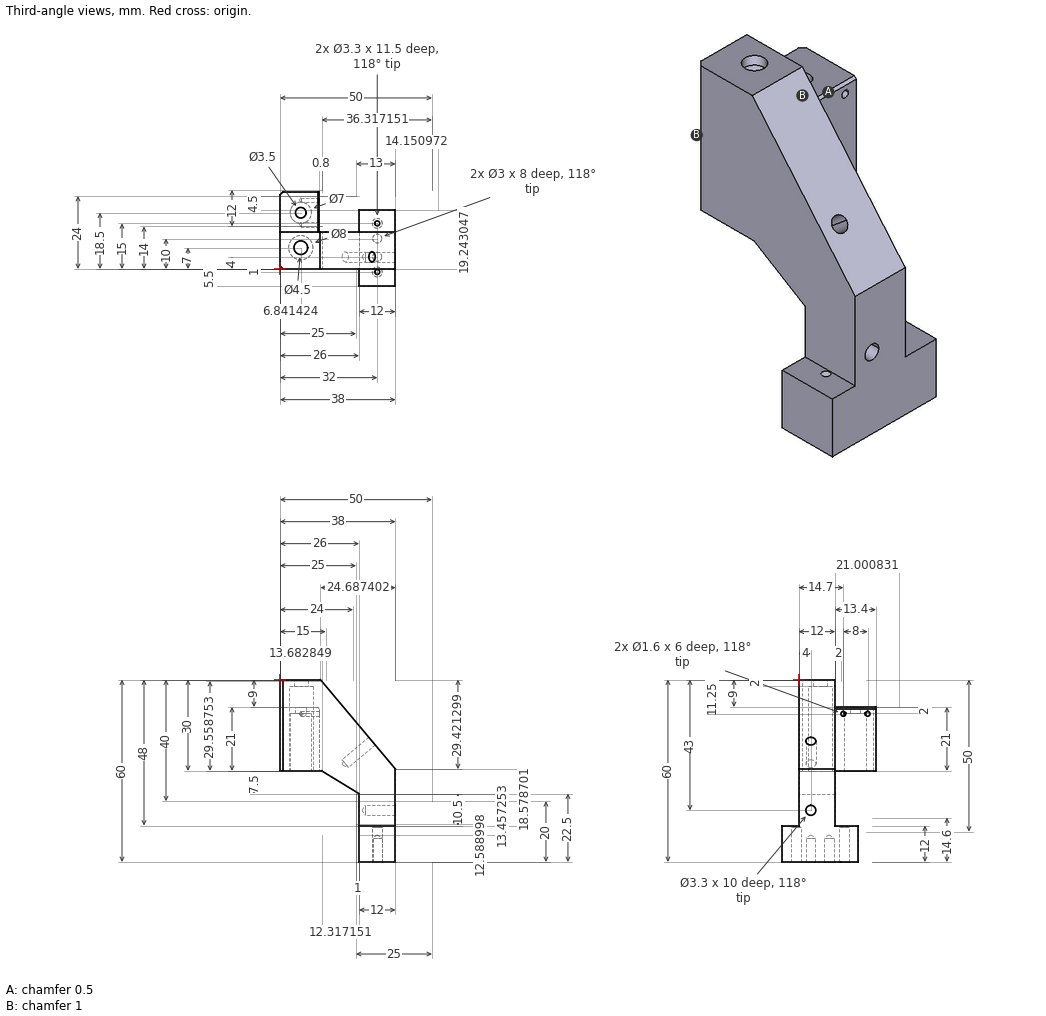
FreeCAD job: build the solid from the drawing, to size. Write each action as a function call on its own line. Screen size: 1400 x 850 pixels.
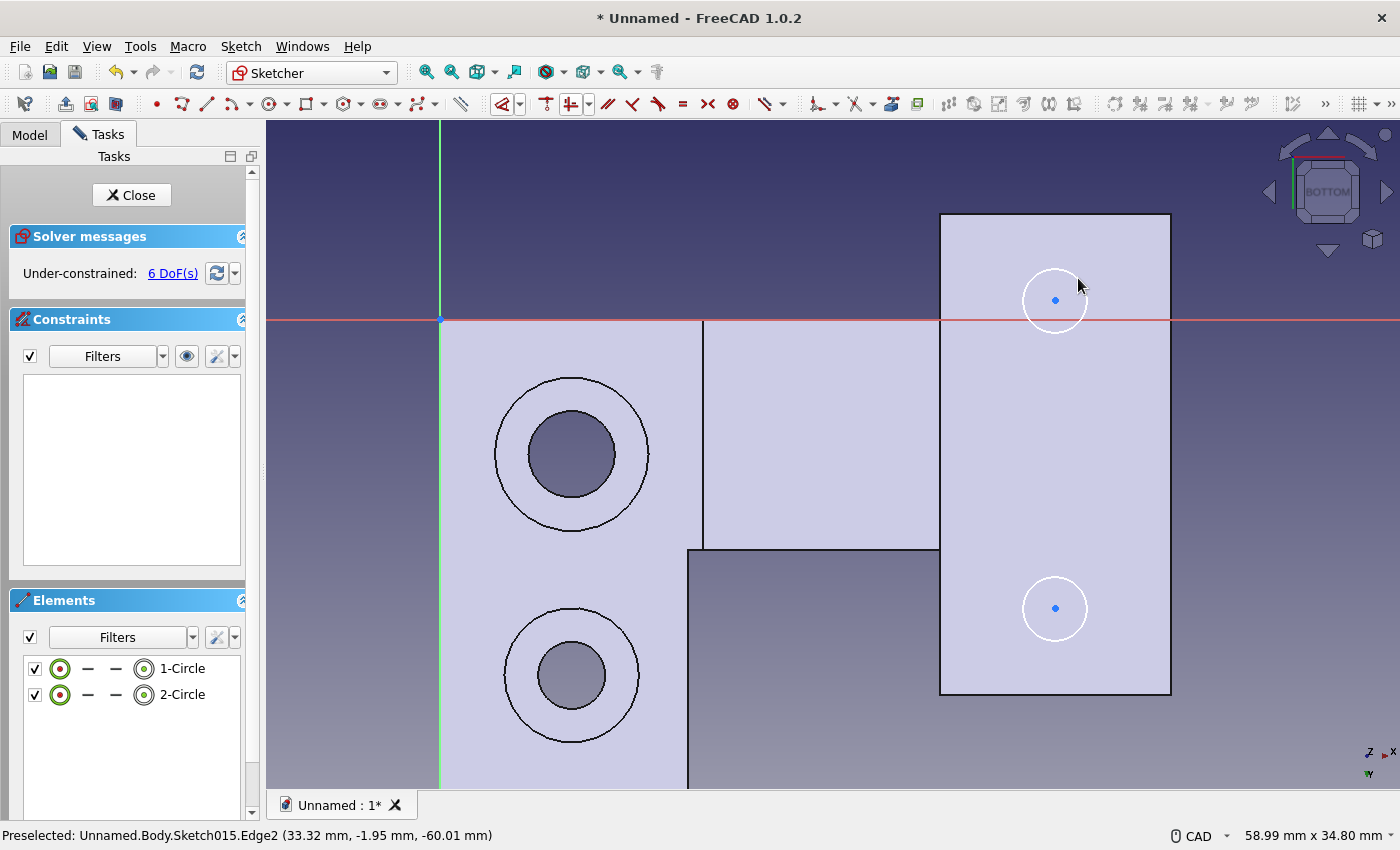
click(1077, 586)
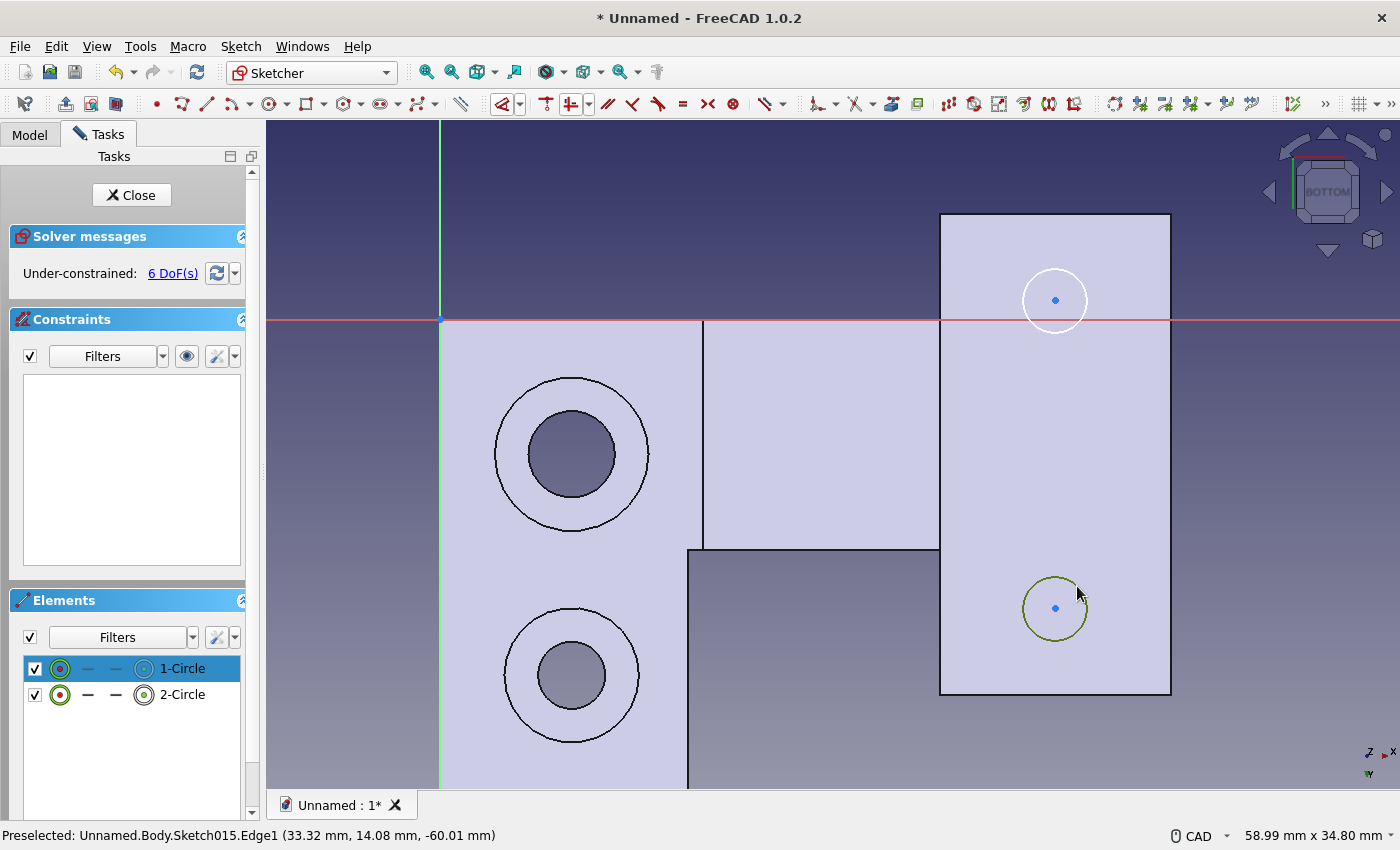
click(1077, 278)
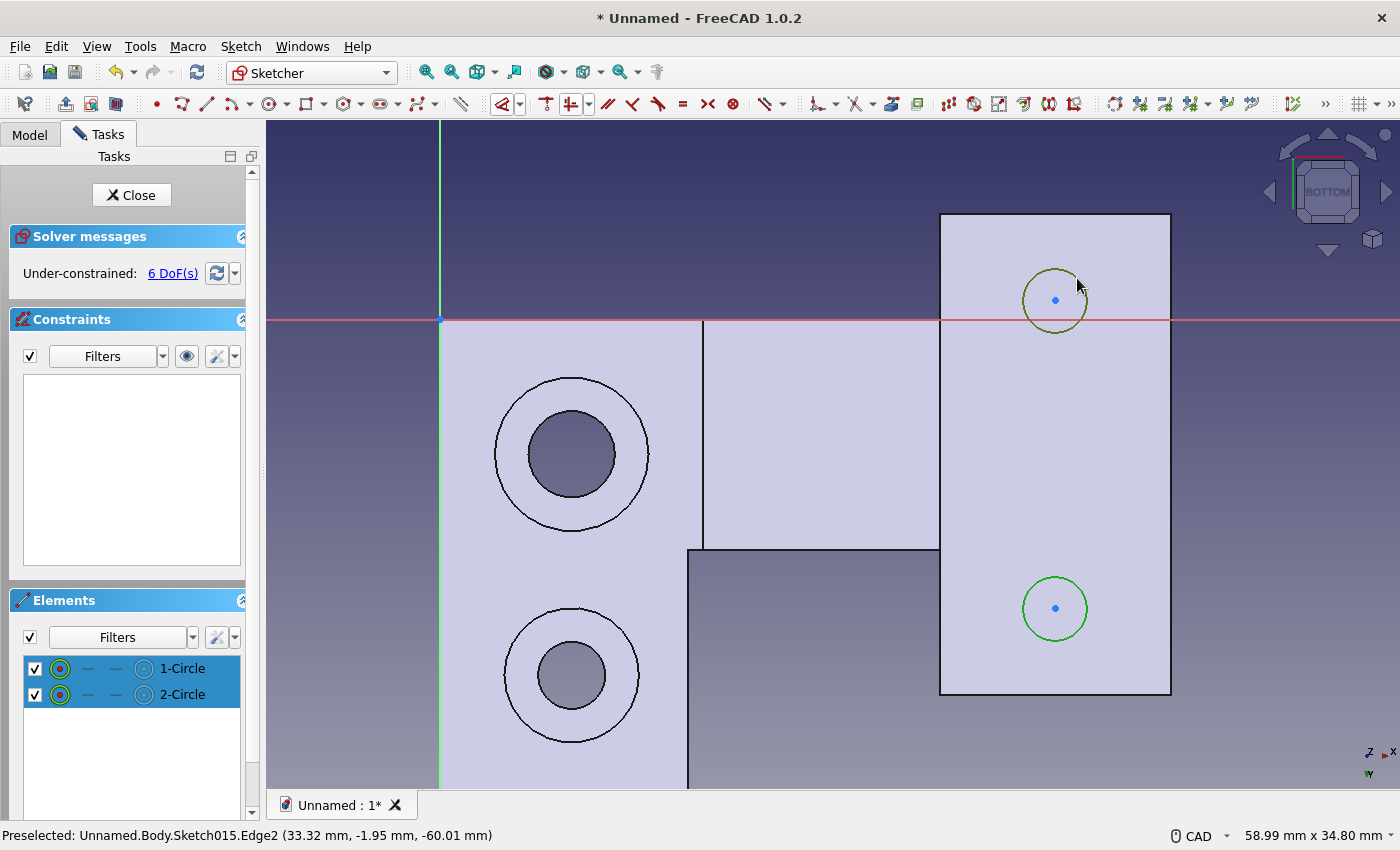
click(683, 104)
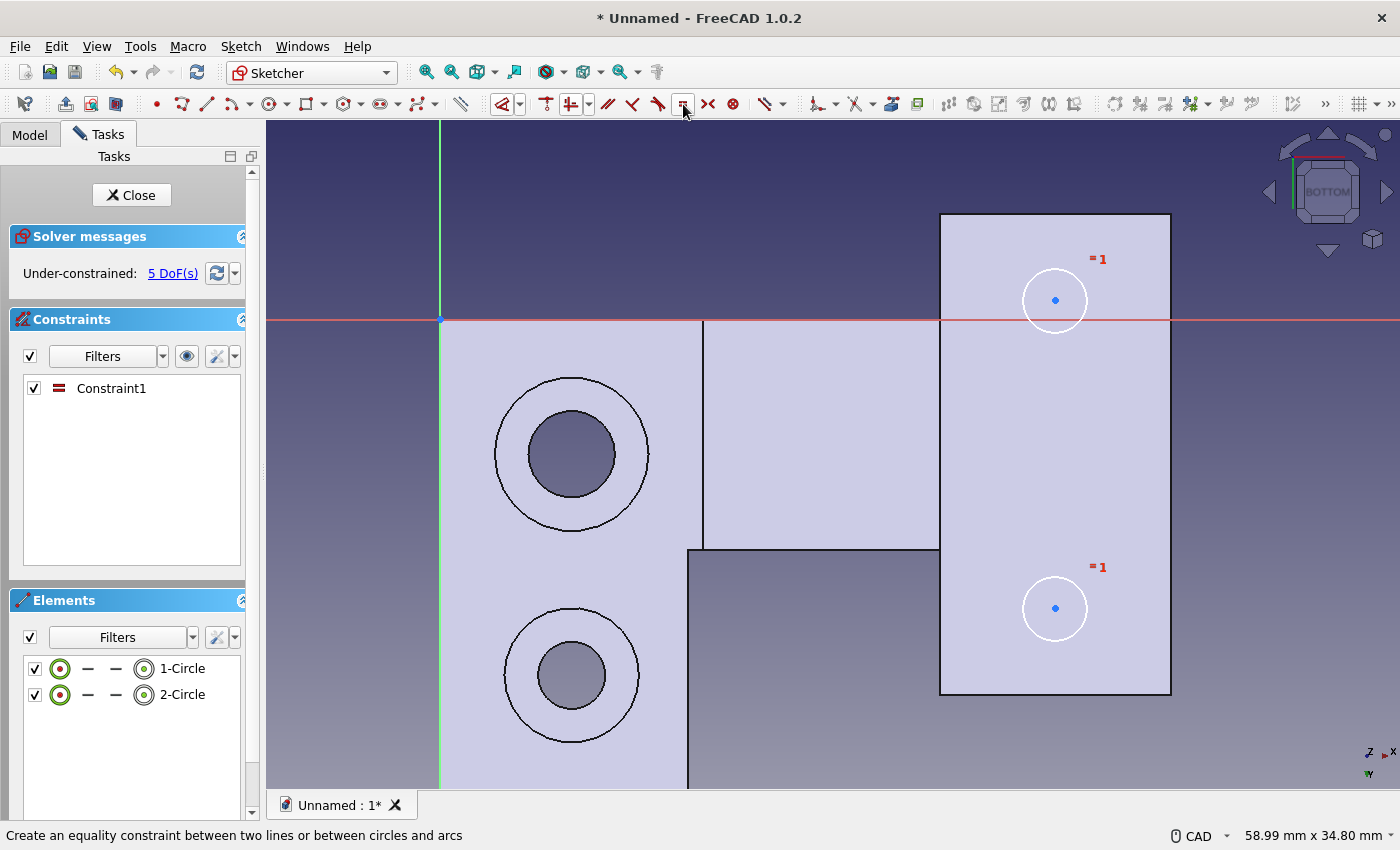
click(1055, 609)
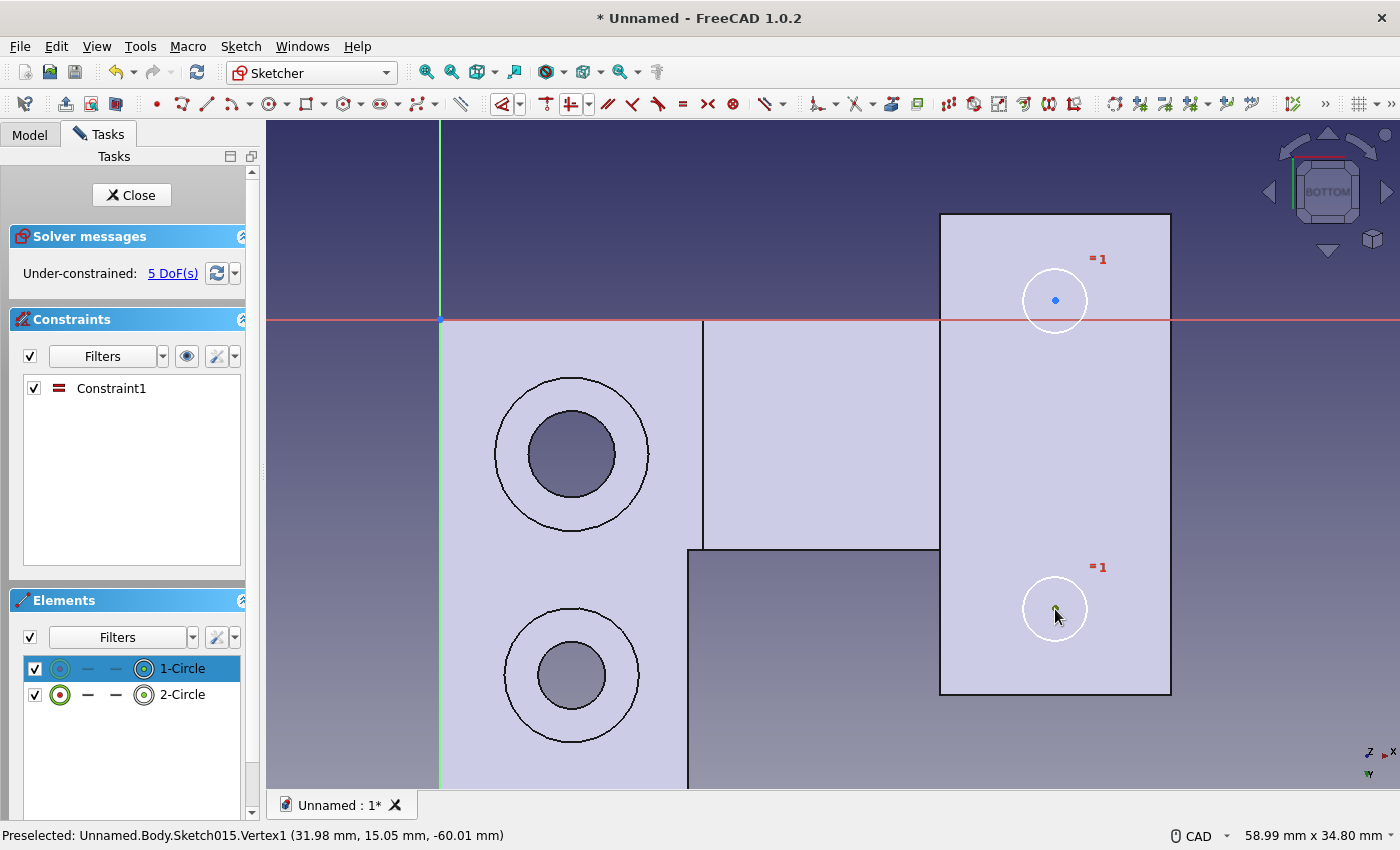
click(1055, 301)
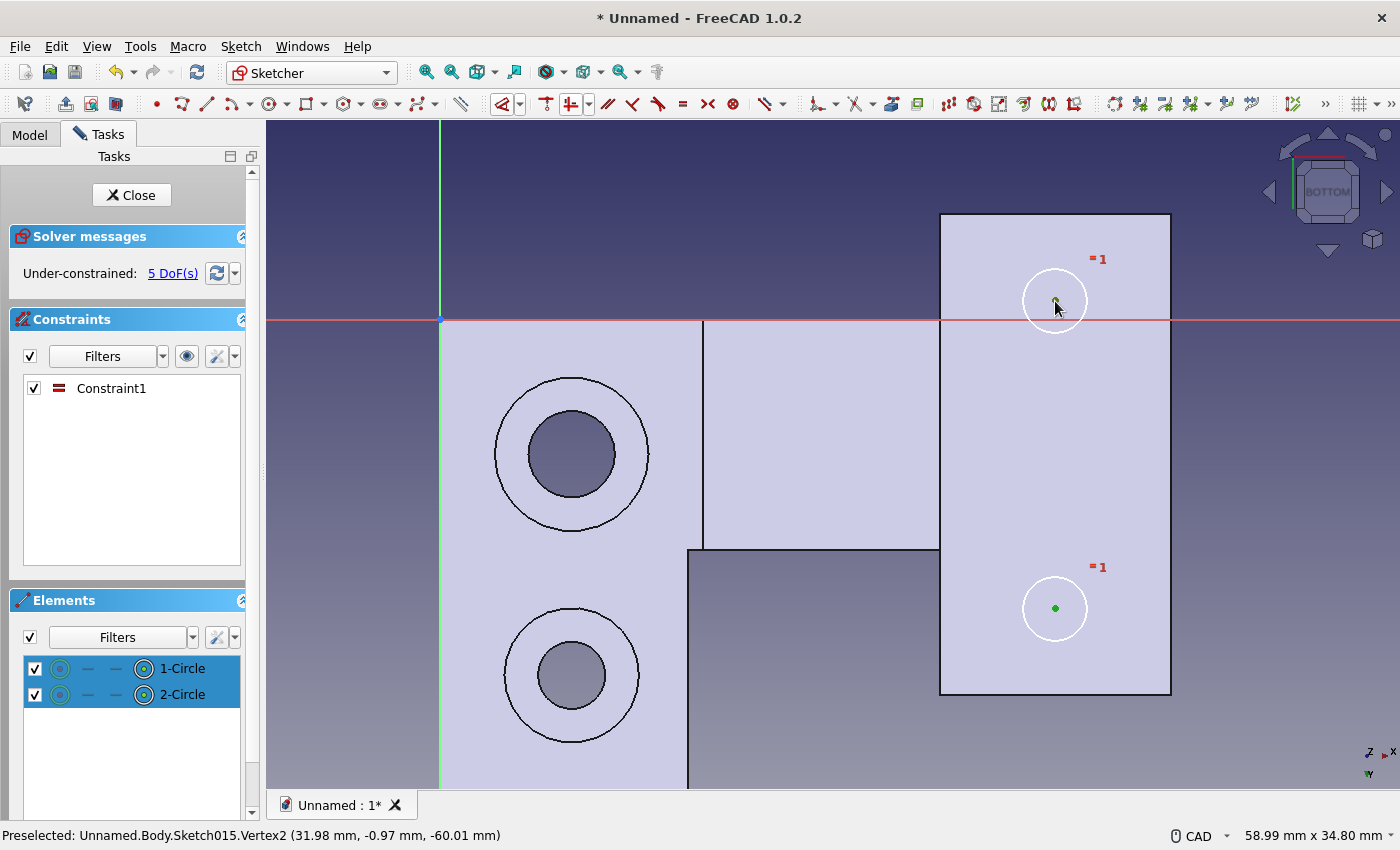
click(588, 104)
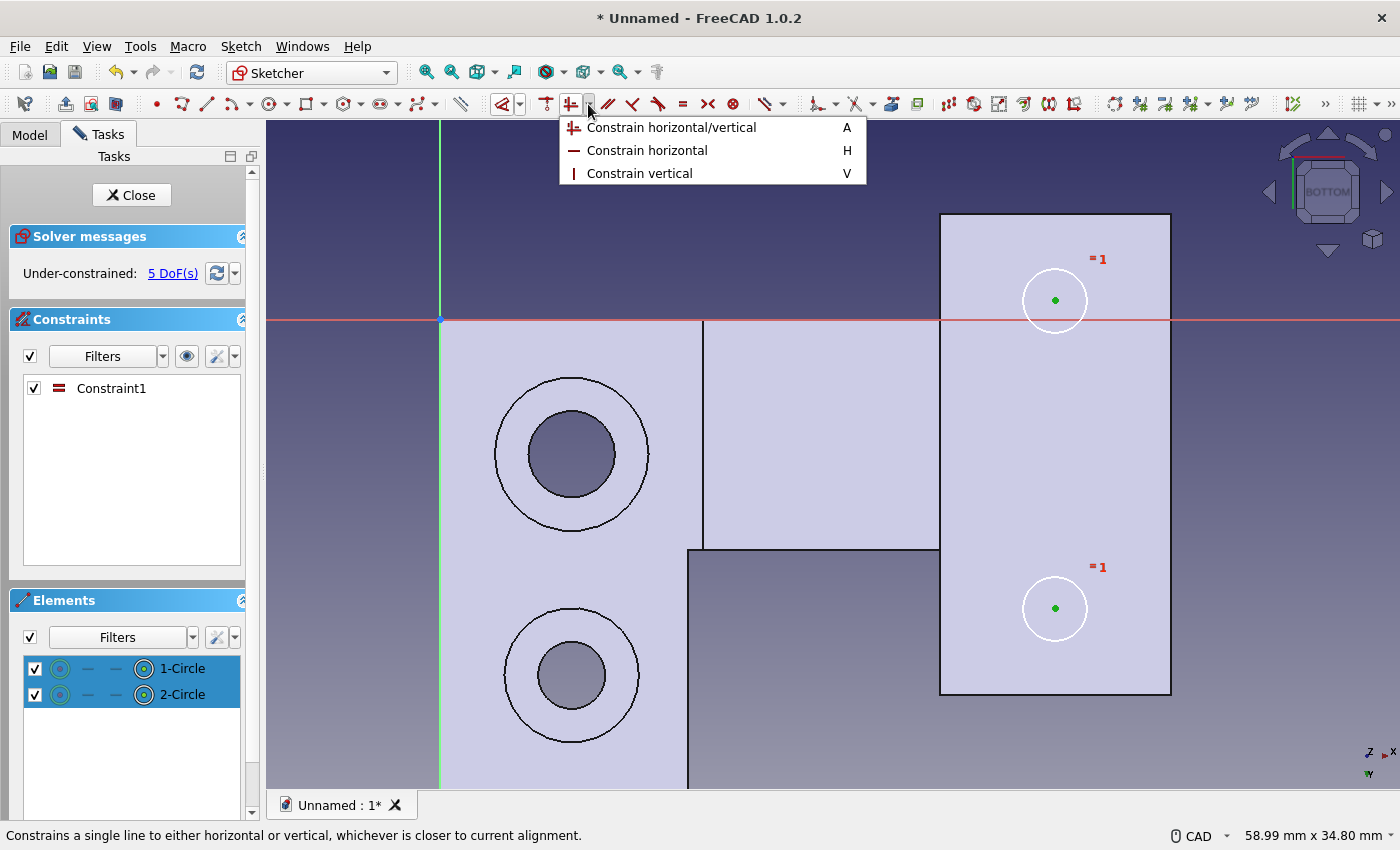
click(713, 174)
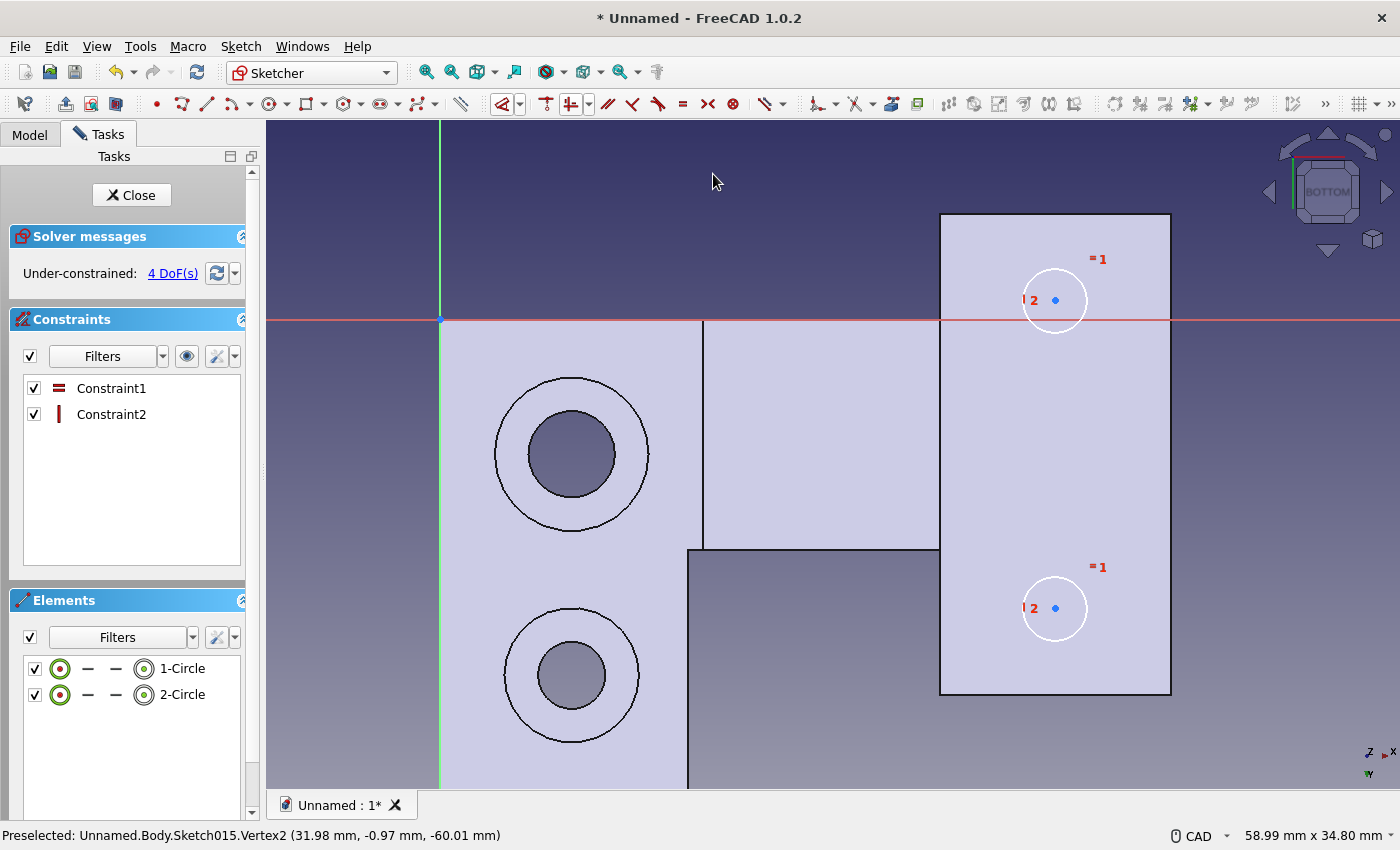
click(1077, 586)